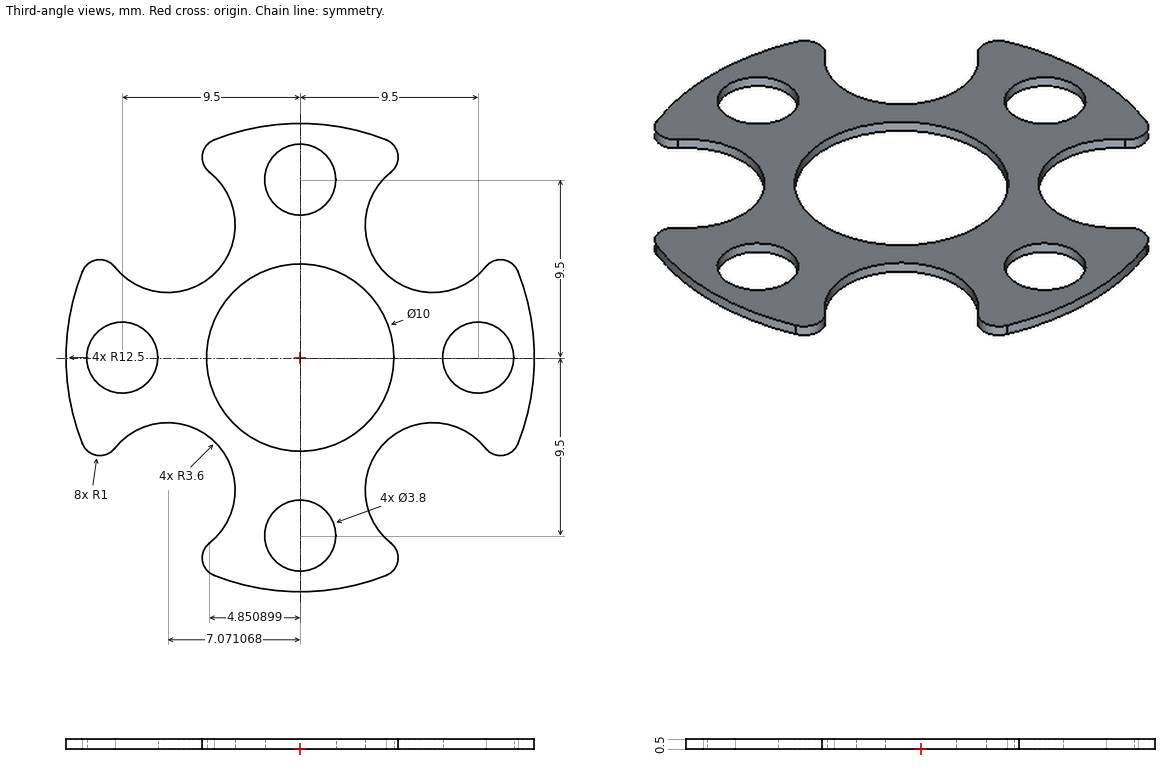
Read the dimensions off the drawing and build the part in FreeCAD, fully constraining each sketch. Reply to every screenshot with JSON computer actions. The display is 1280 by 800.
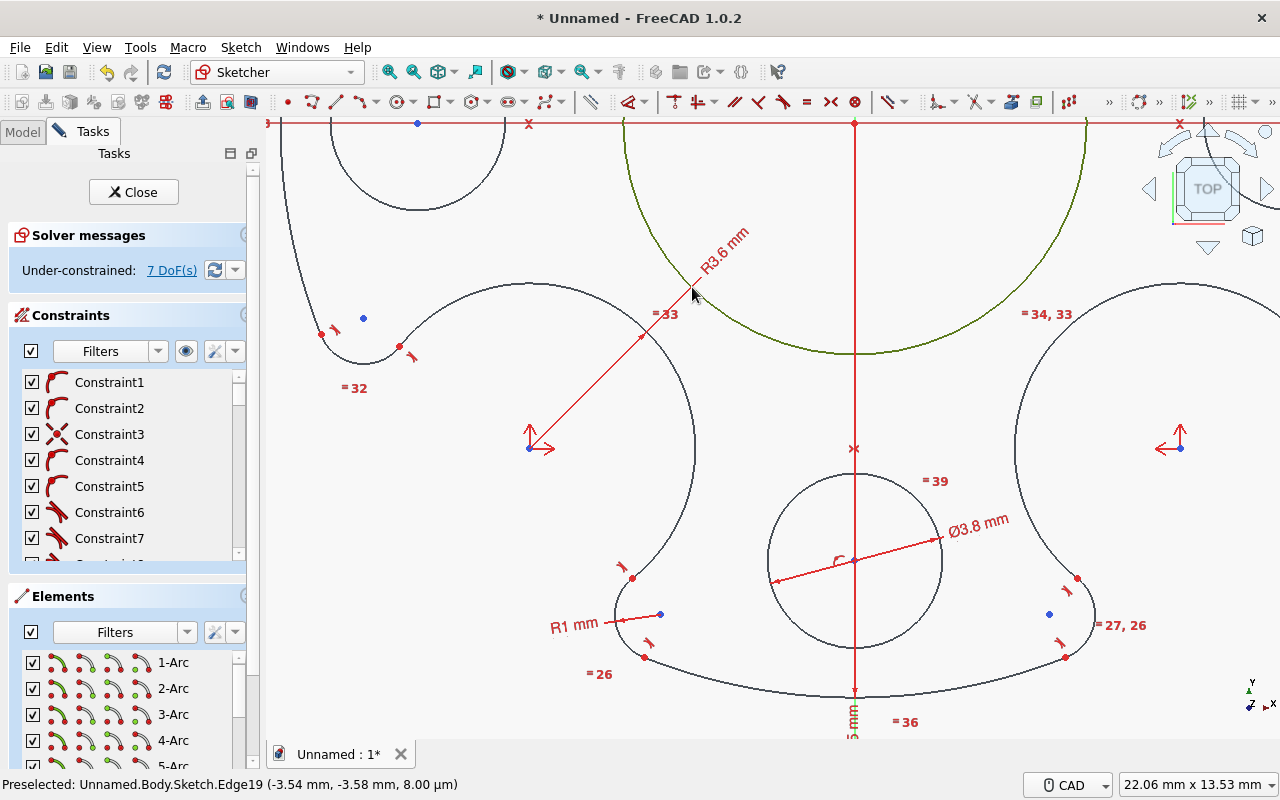
{"action": "key", "text": "k o"}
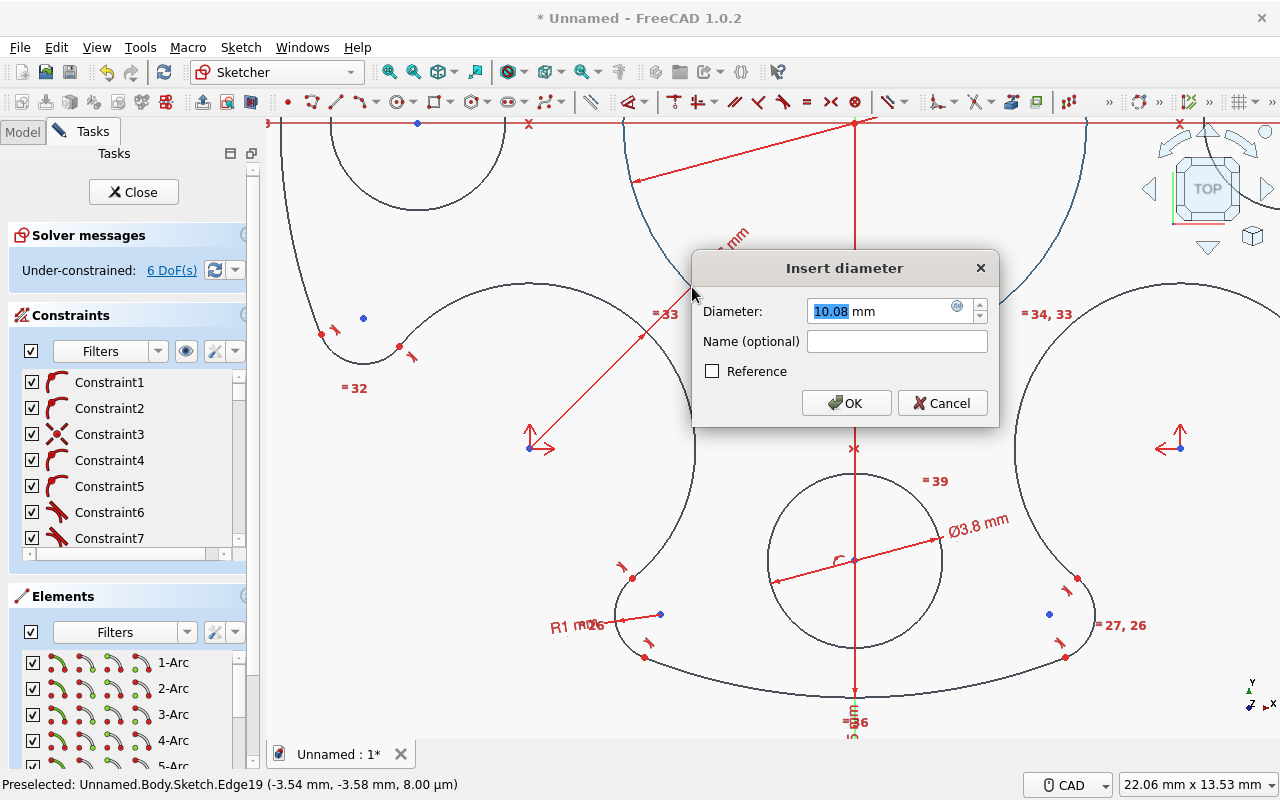
{"action": "type", "text": "10"}
{"action": "key", "text": "Return"}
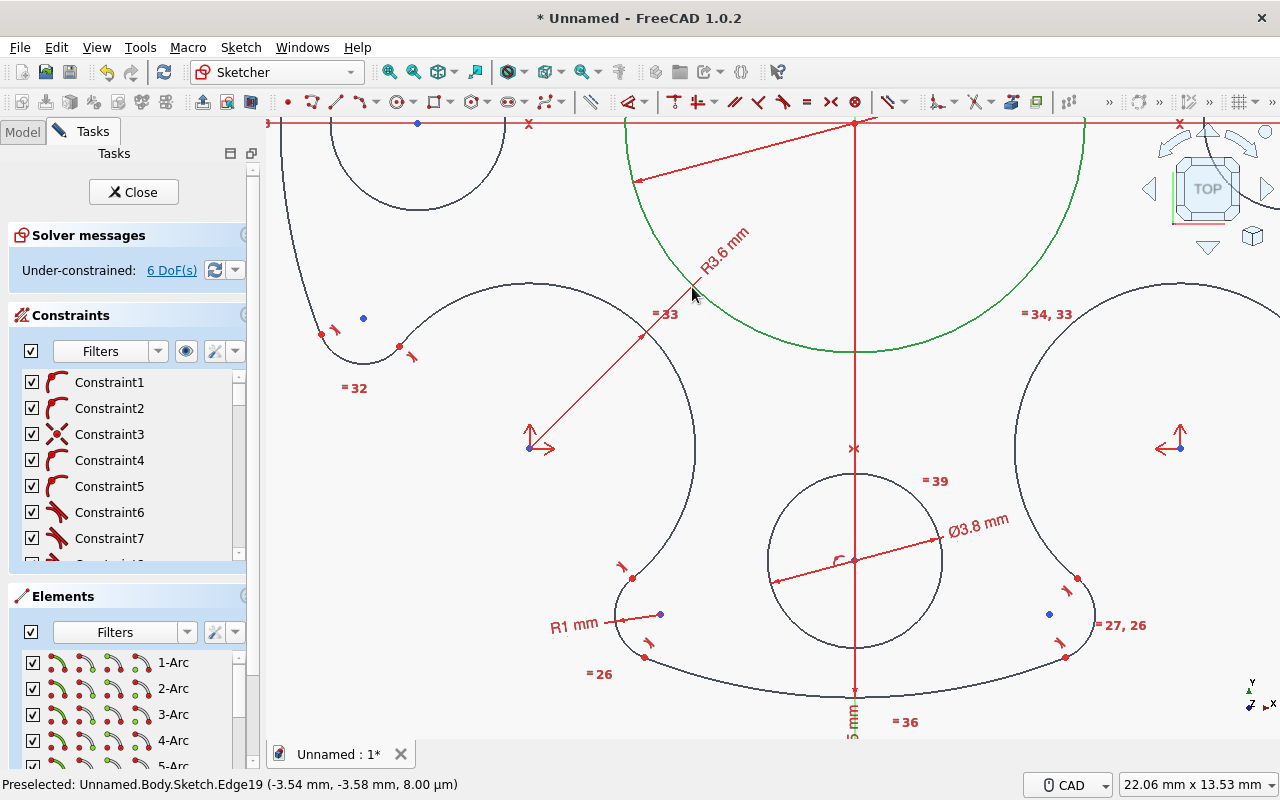
{"action": "left_click", "coordinate": [855, 561]}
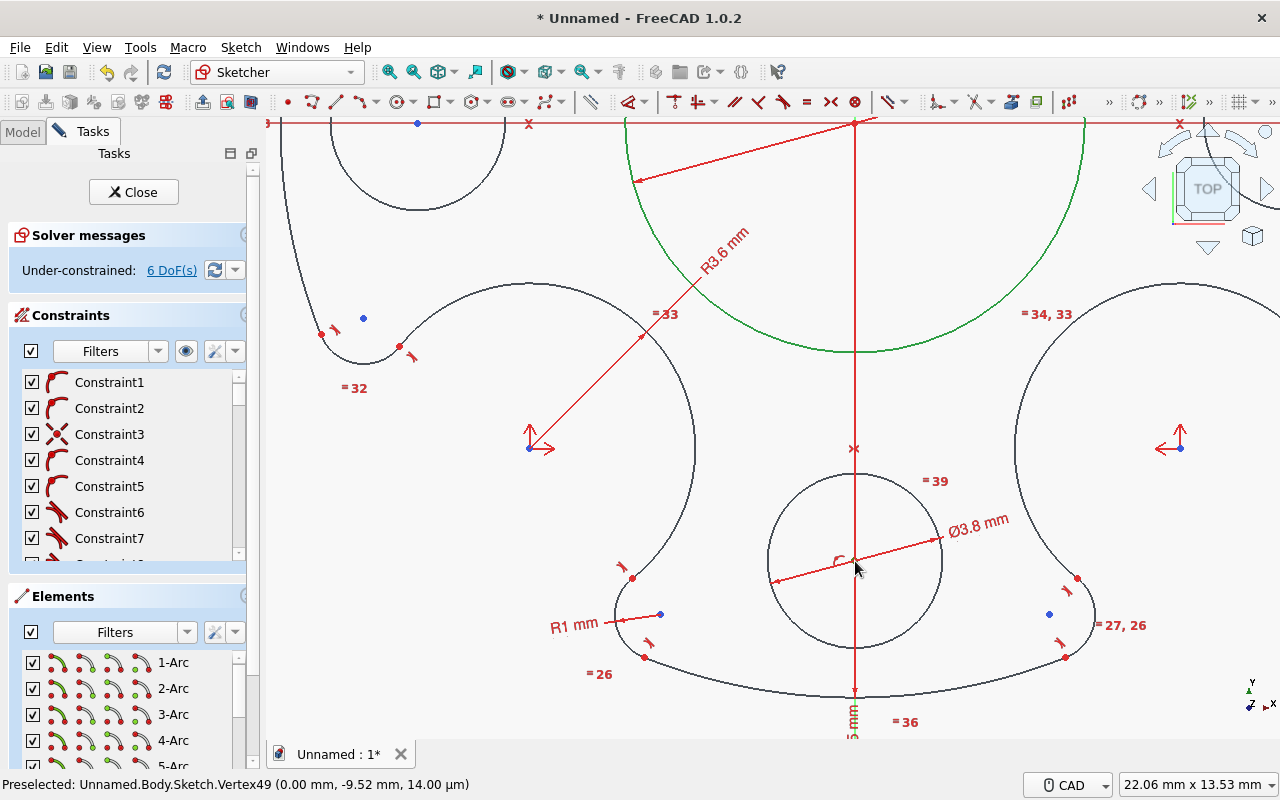
{"action": "key", "text": "i"}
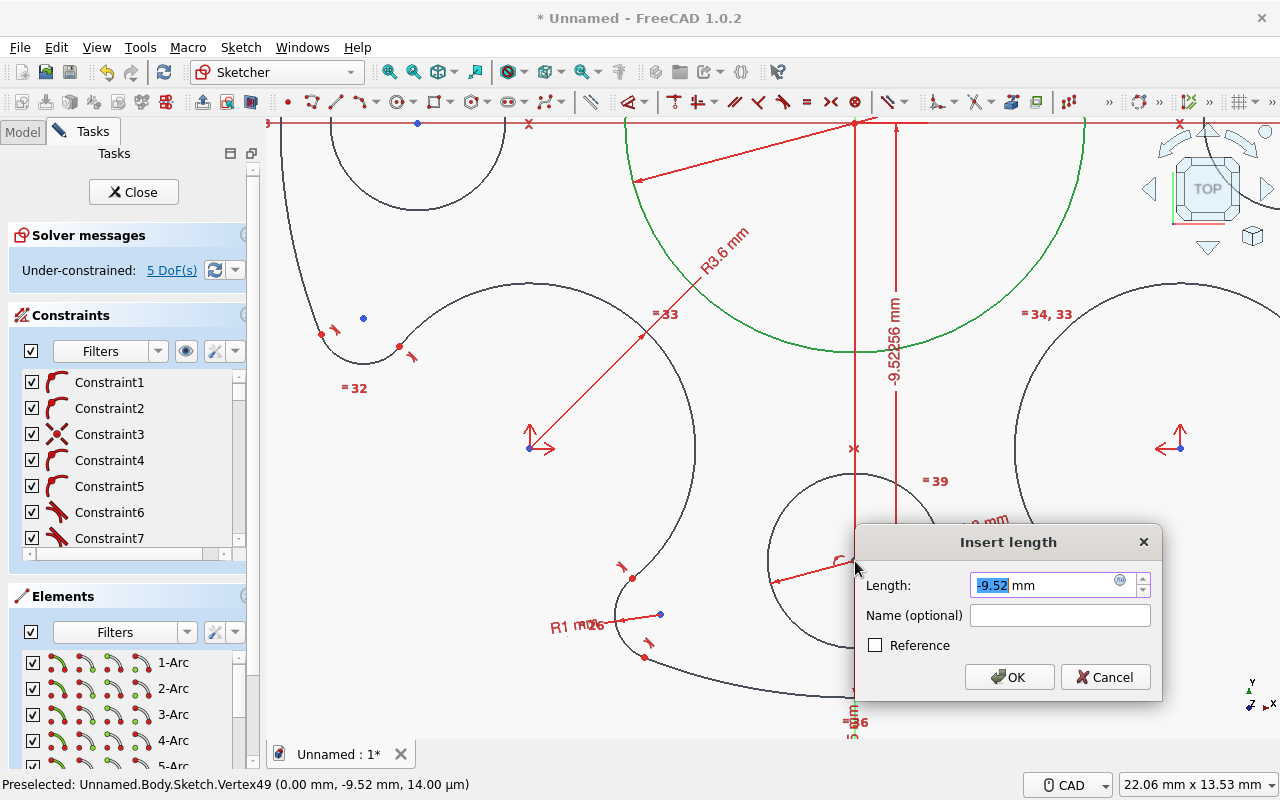
{"action": "type", "text": "-9.5"}
{"action": "key", "text": "Return"}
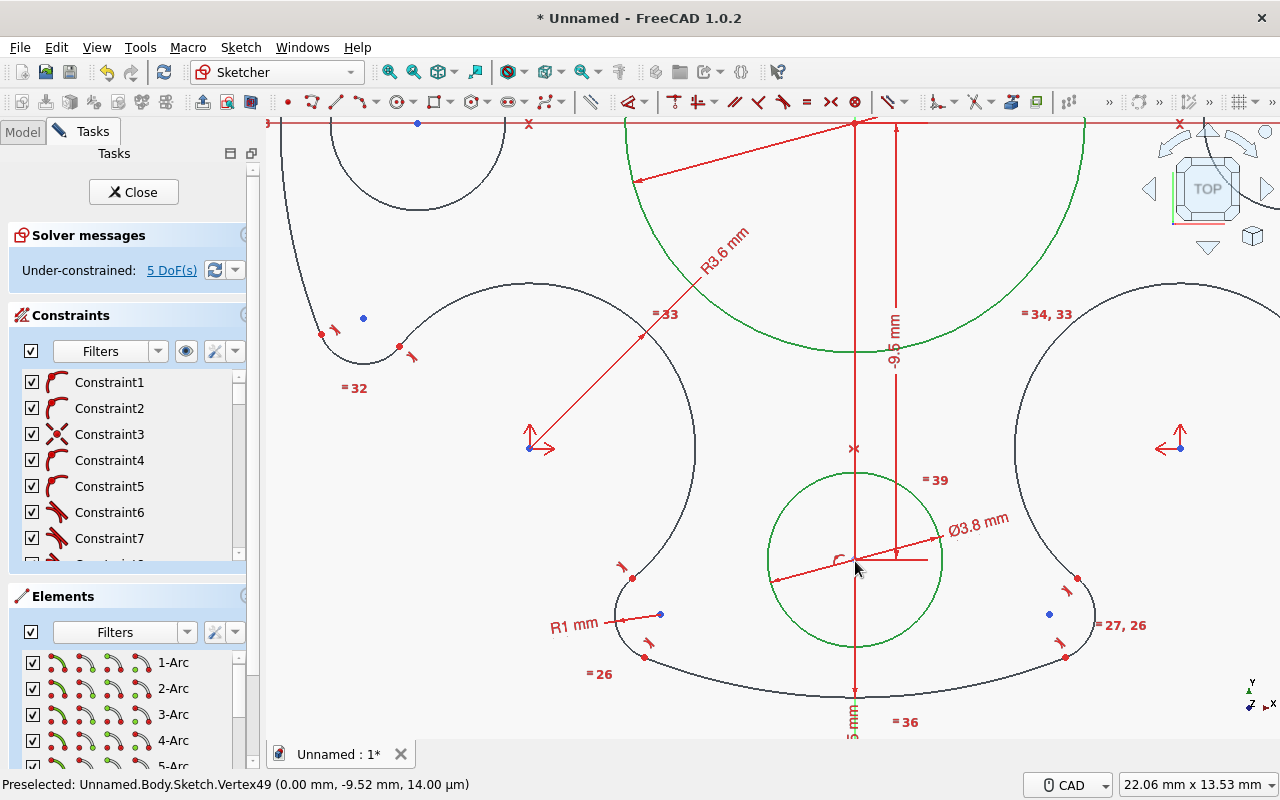
{"action": "scroll", "coordinate": [617, 605], "scroll_direction": "down", "scroll_amount": 5}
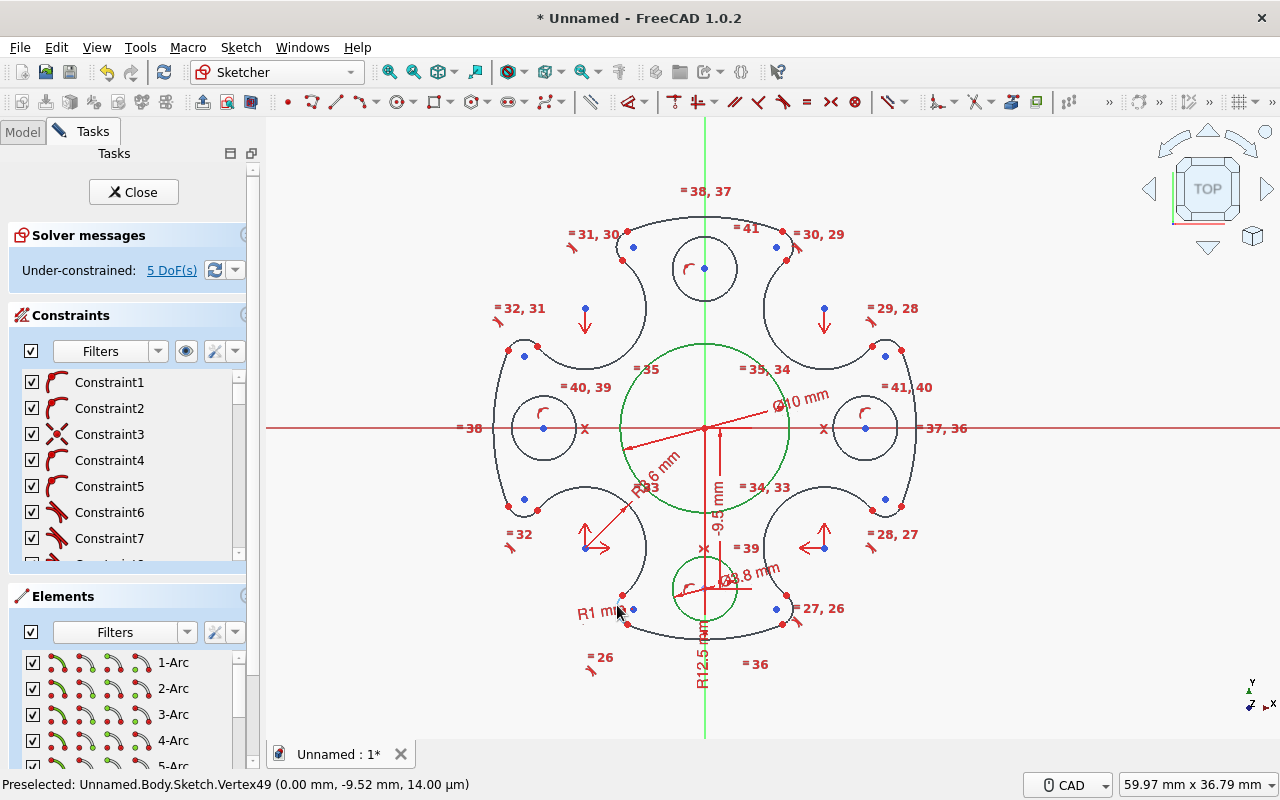
{"action": "left_click", "coordinate": [544, 428]}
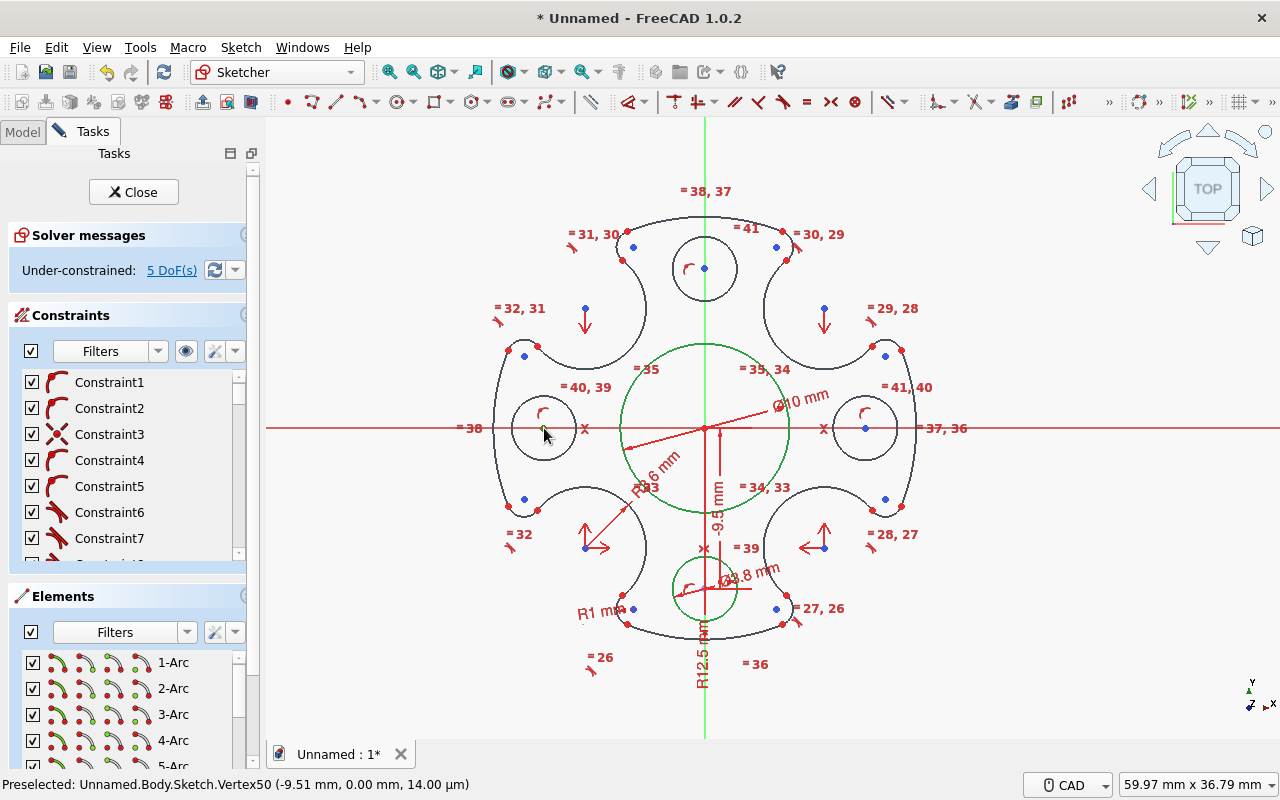
{"action": "left_click", "coordinate": [646, 102]}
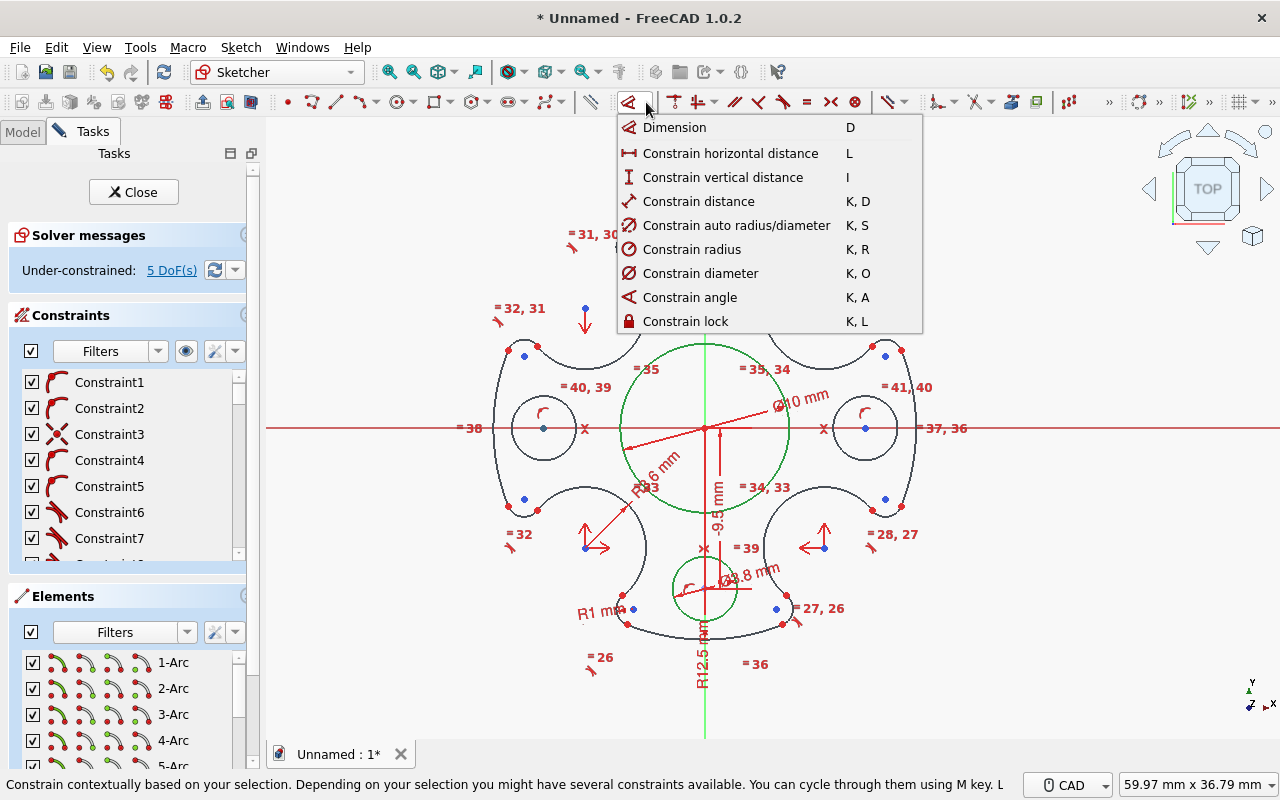
{"action": "left_click", "coordinate": [770, 153]}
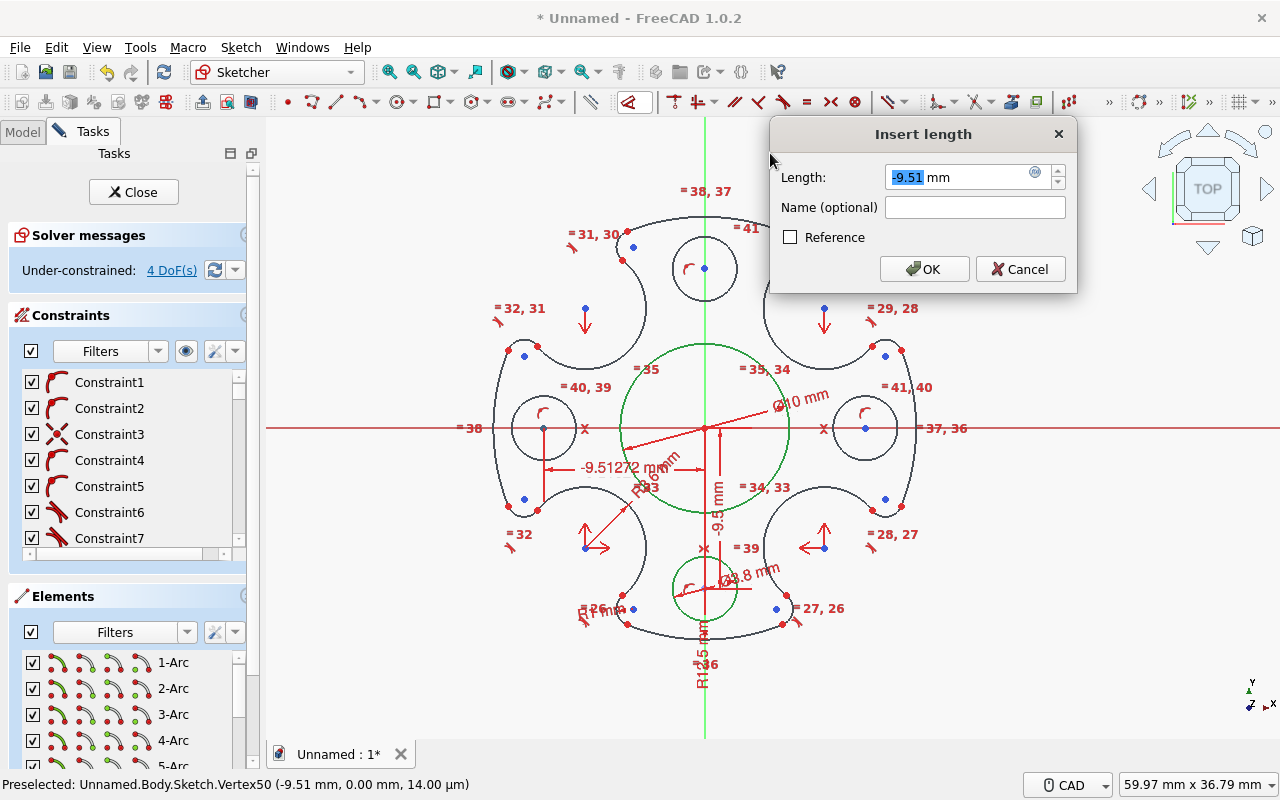
{"action": "type", "text": "-9.5"}
{"action": "key", "text": "Return"}